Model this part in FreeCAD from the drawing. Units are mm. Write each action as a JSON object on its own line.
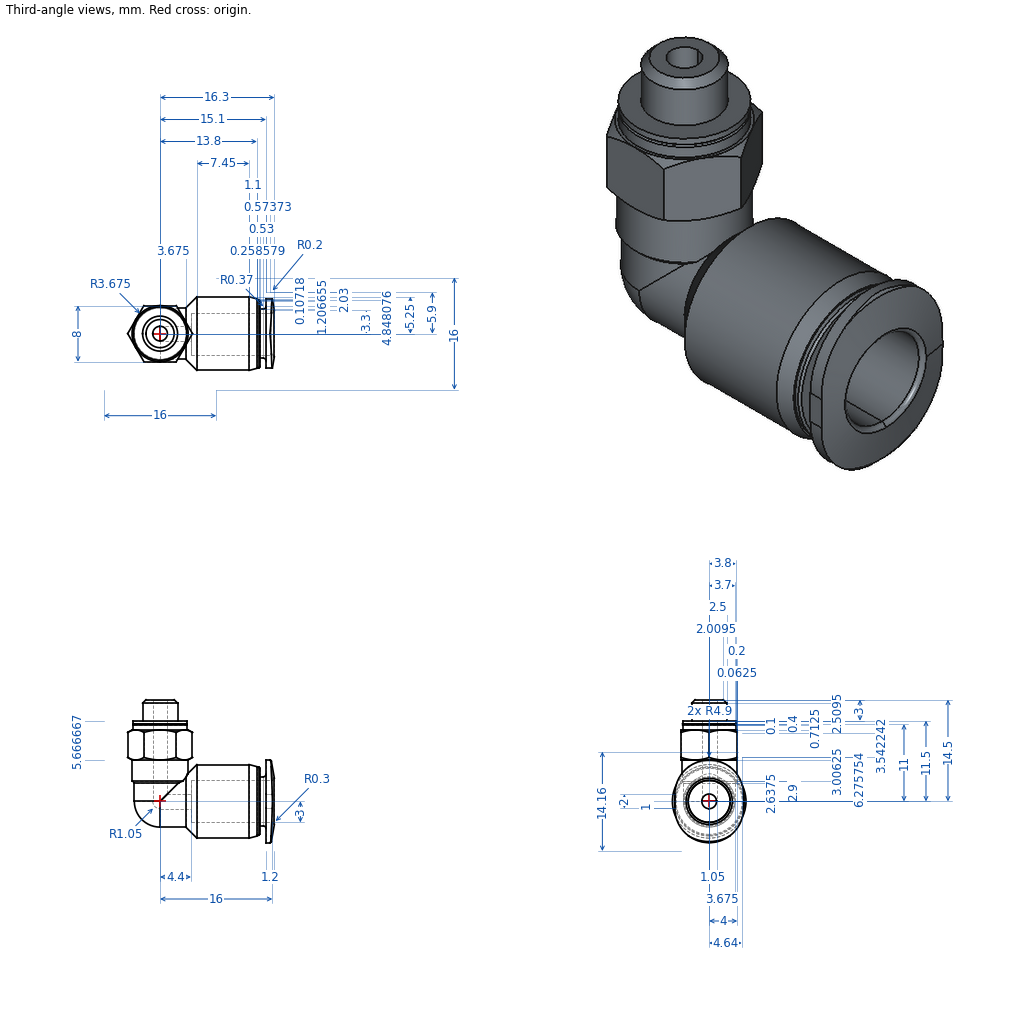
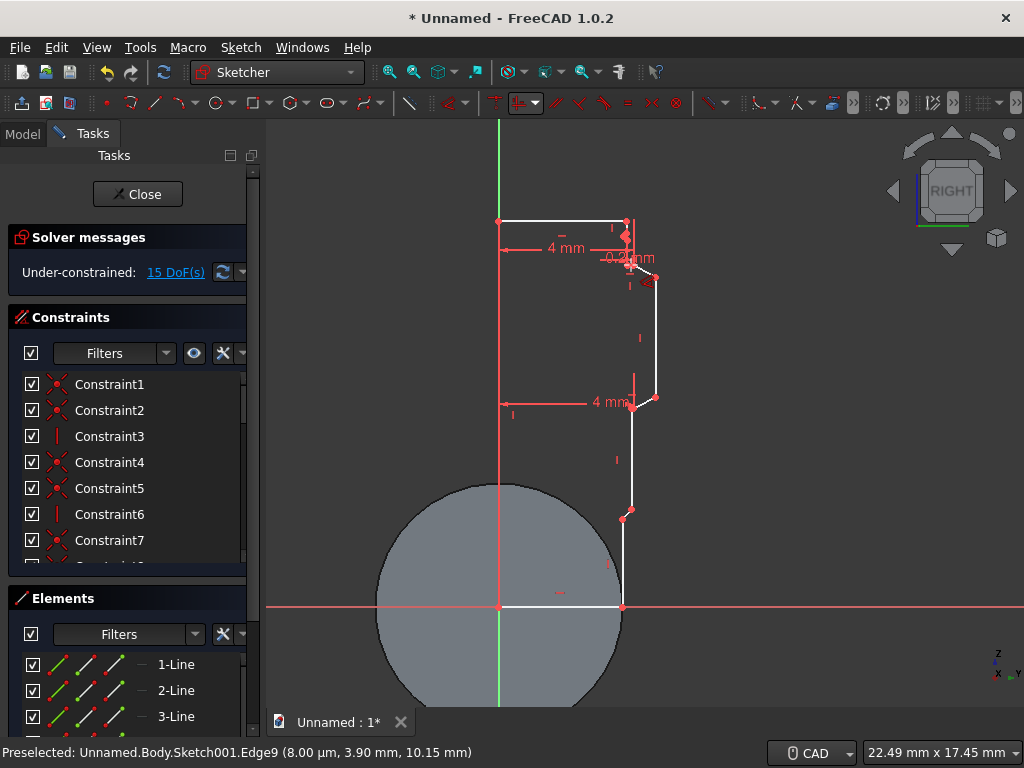
{"action": "scroll", "coordinate": [627, 230], "scroll_direction": "up", "scroll_amount": 7}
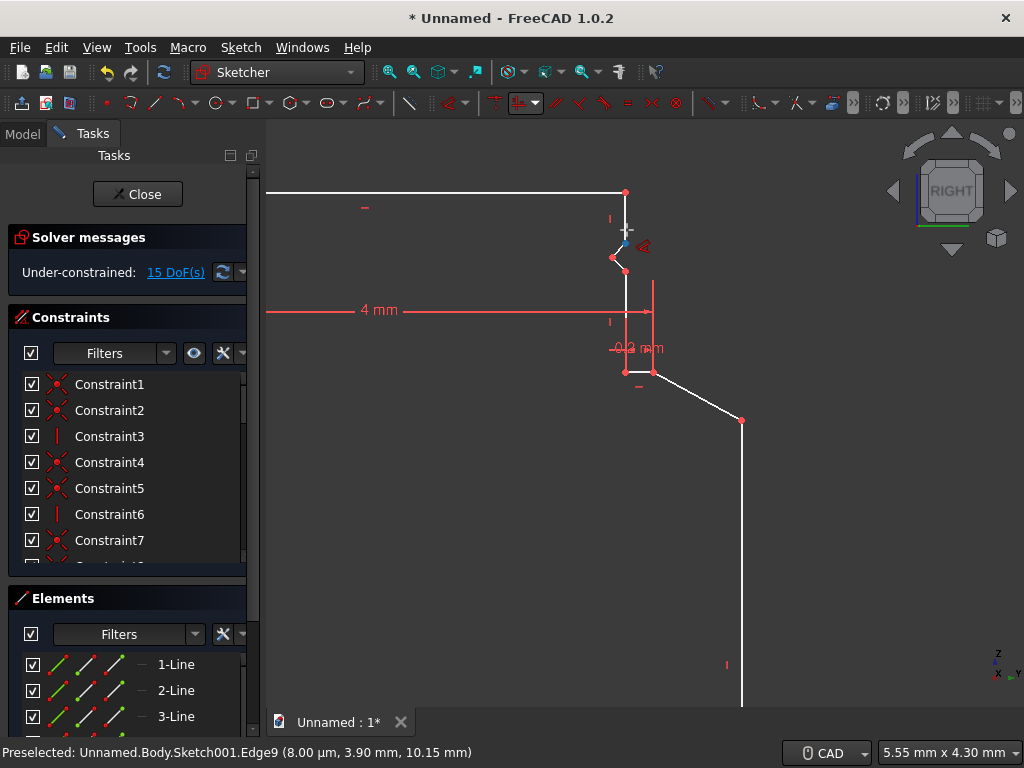
{"action": "left_click", "coordinate": [625, 228]}
{"action": "left_click", "coordinate": [659, 218]}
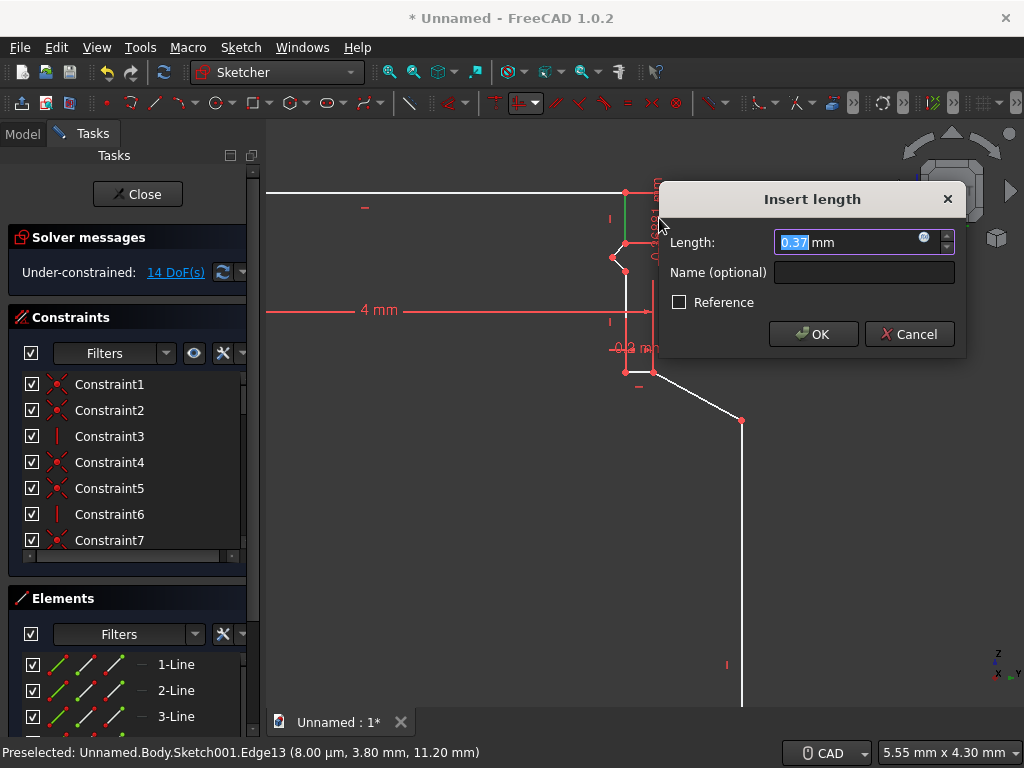
{"action": "type", "text": "0.4"}
{"action": "key", "text": "Return"}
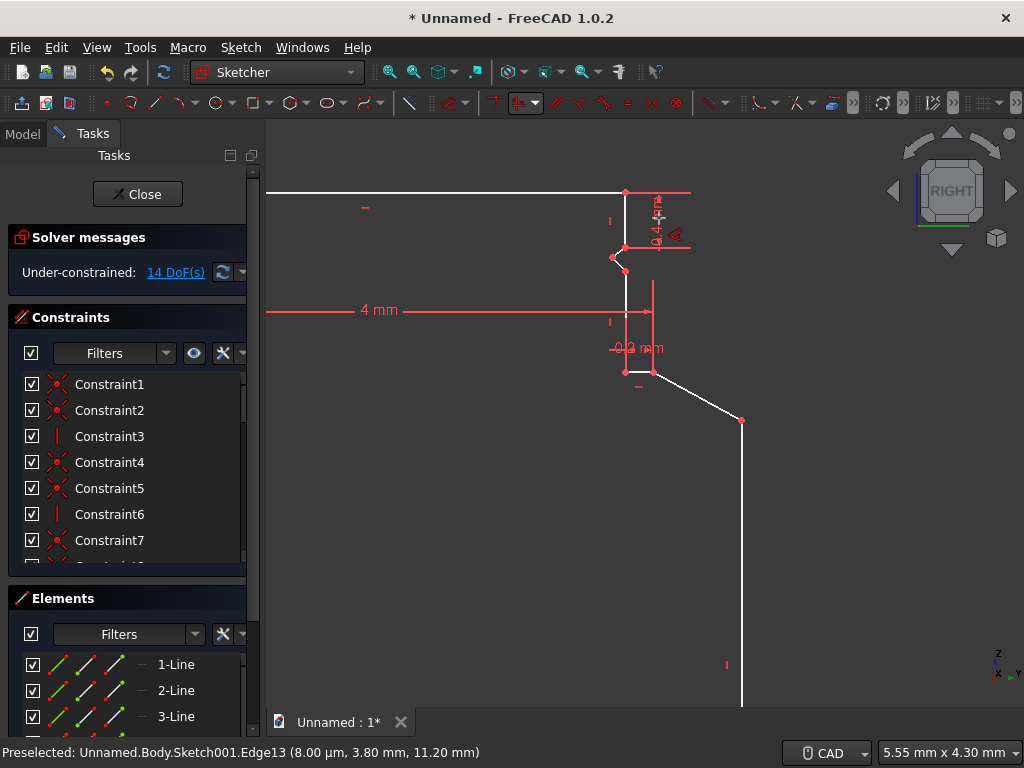
{"action": "scroll", "coordinate": [627, 230], "scroll_direction": "down", "scroll_amount": 7}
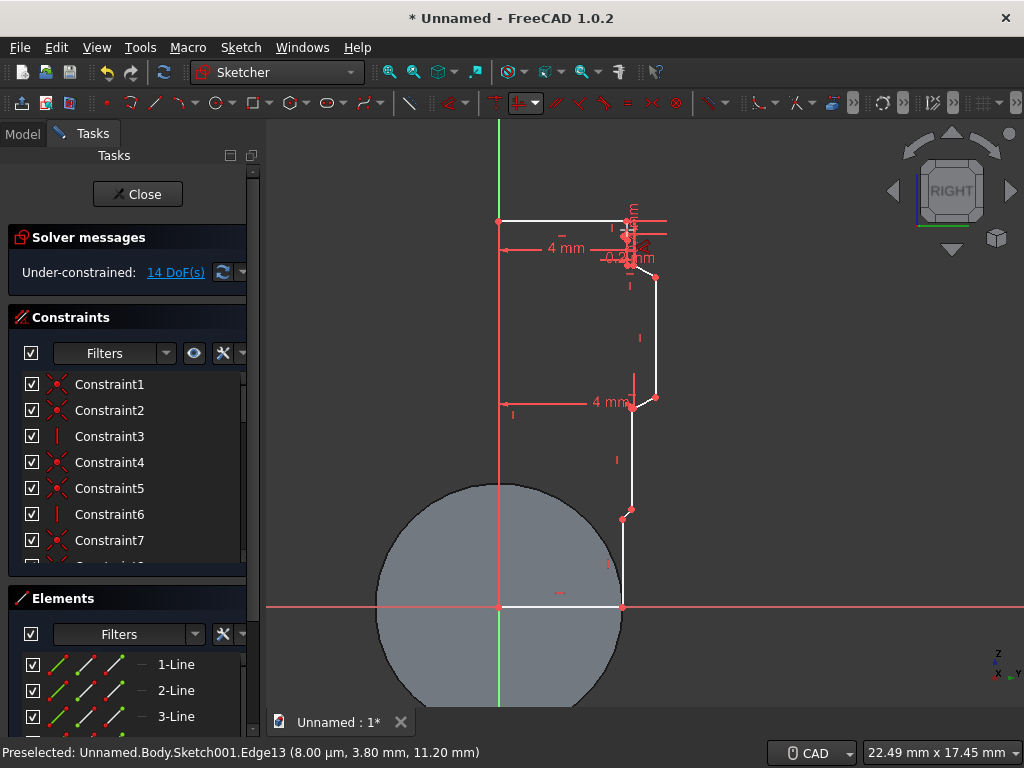
{"action": "left_click", "coordinate": [589, 221]}
{"action": "left_click", "coordinate": [563, 187]}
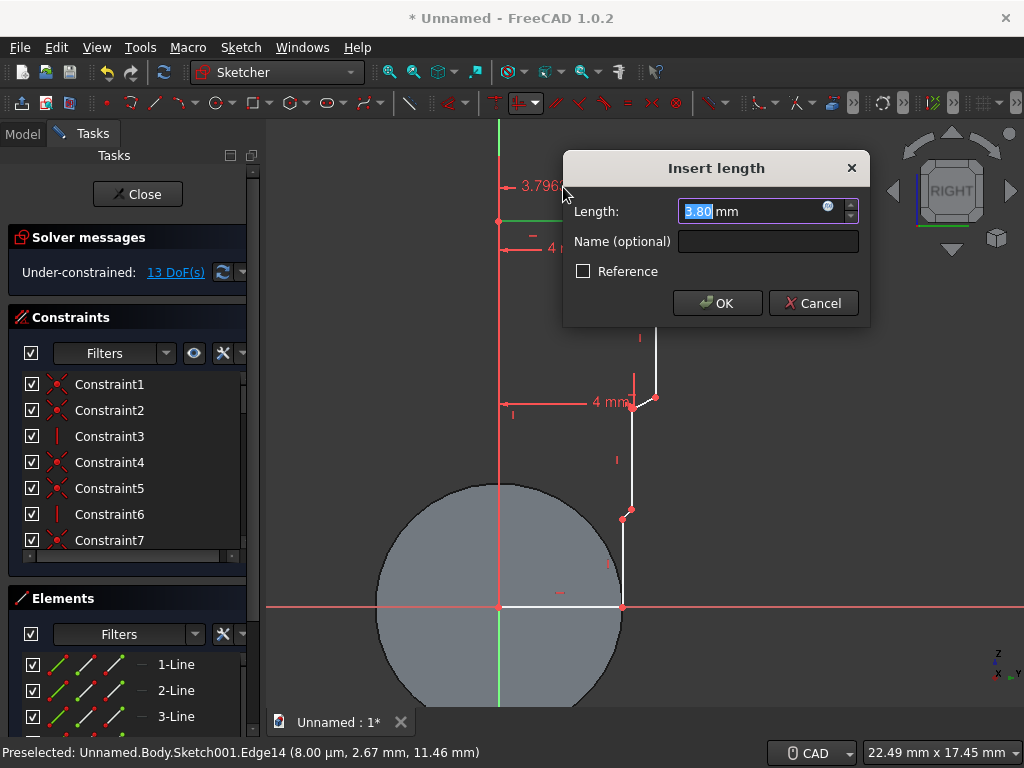
{"action": "type", "text": "3.8"}
{"action": "key", "text": "Return"}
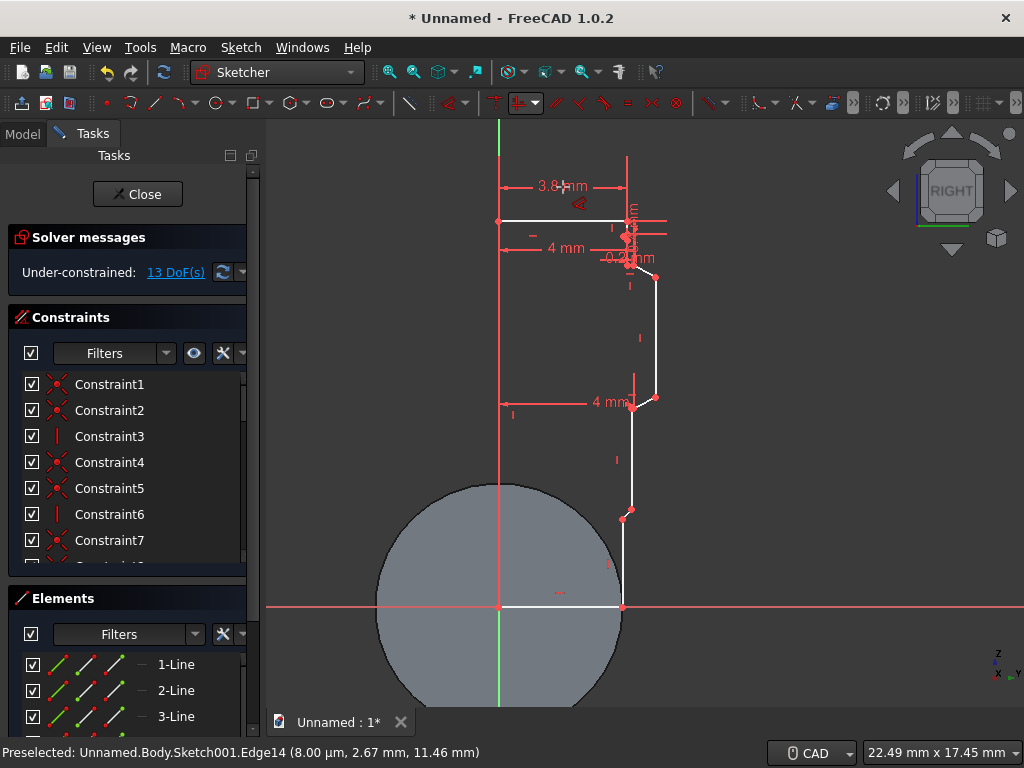
{"action": "scroll", "coordinate": [624, 237], "scroll_direction": "up", "scroll_amount": 6}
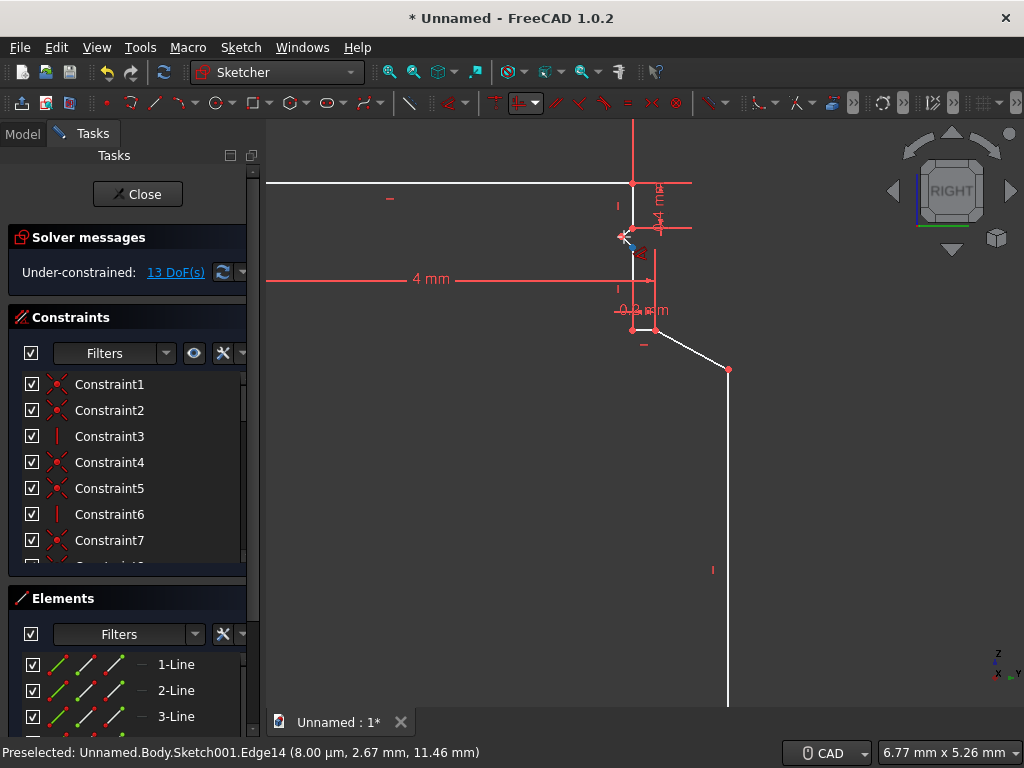
{"action": "left_click", "coordinate": [622, 236]}
{"action": "left_click", "coordinate": [656, 458]}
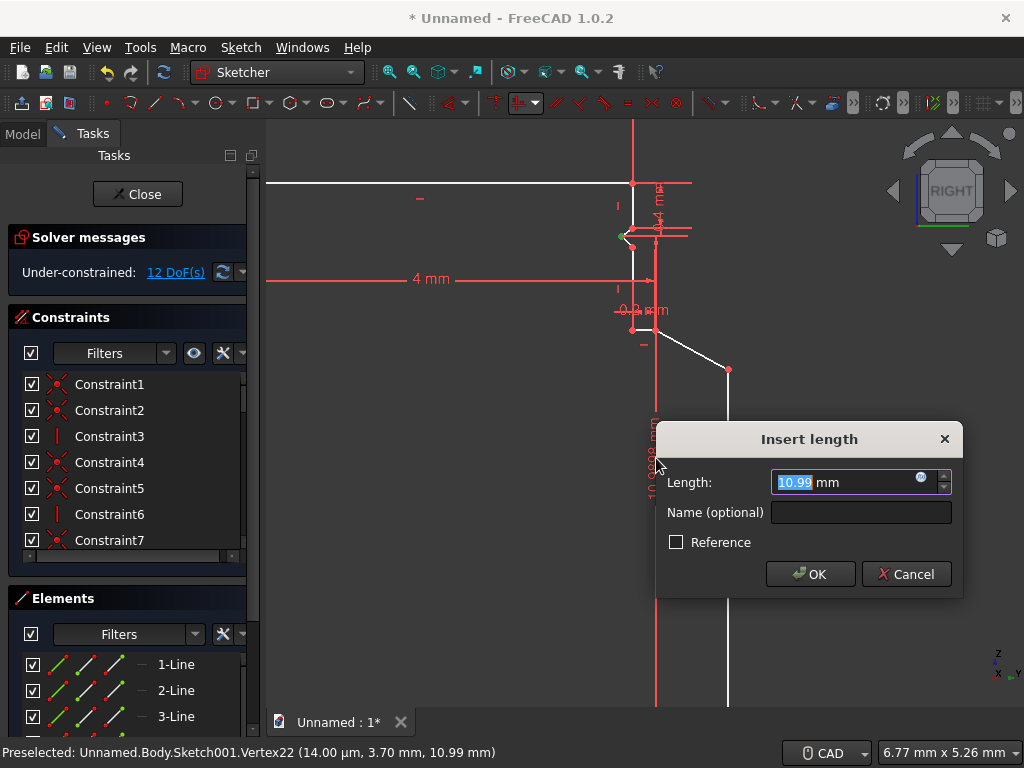
{"action": "type", "text": "11"}
{"action": "key", "text": "Return"}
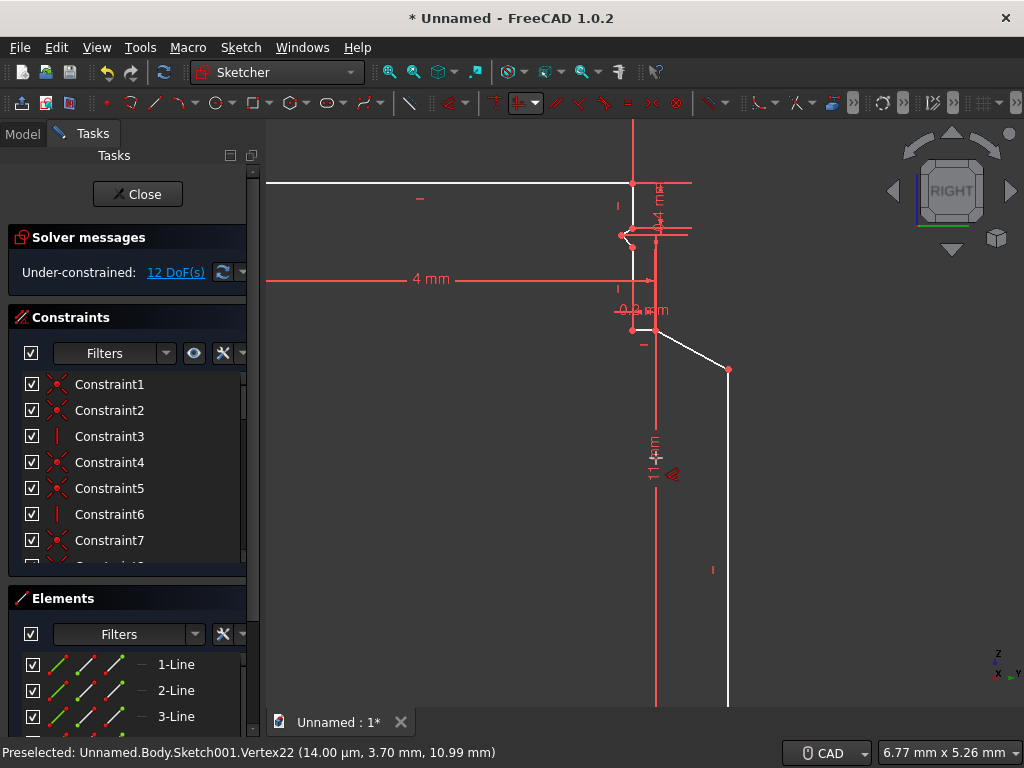
{"action": "scroll", "coordinate": [624, 237], "scroll_direction": "down", "scroll_amount": 6}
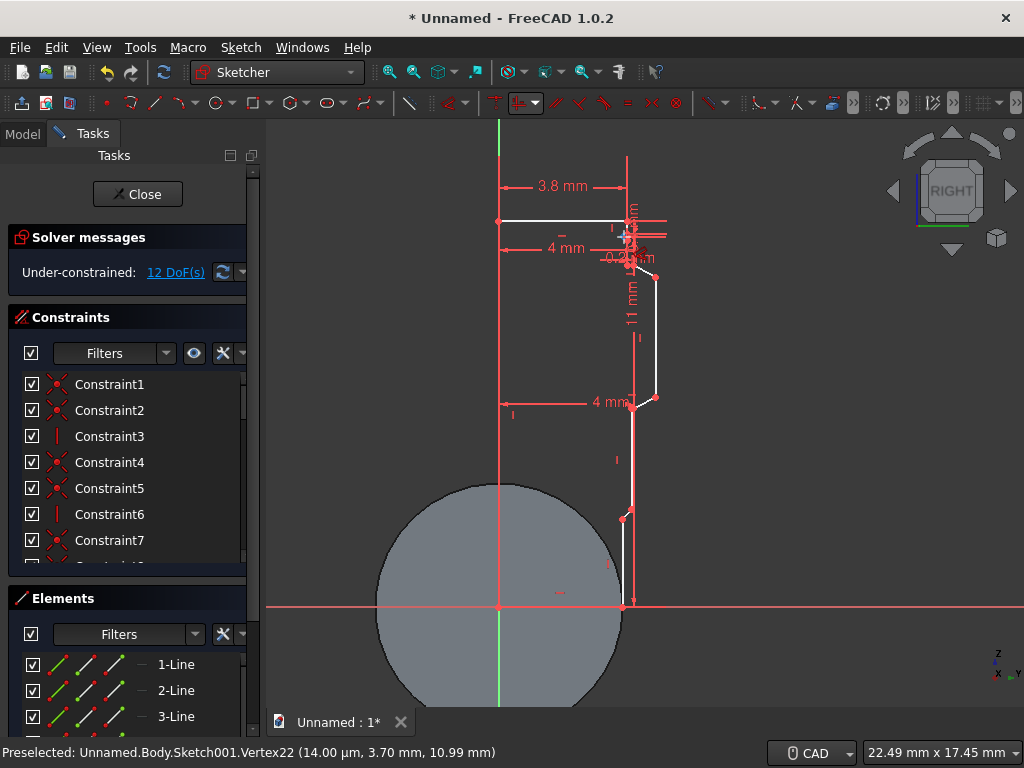
{"action": "left_click", "coordinate": [499, 337]}
{"action": "left_click", "coordinate": [465, 414]}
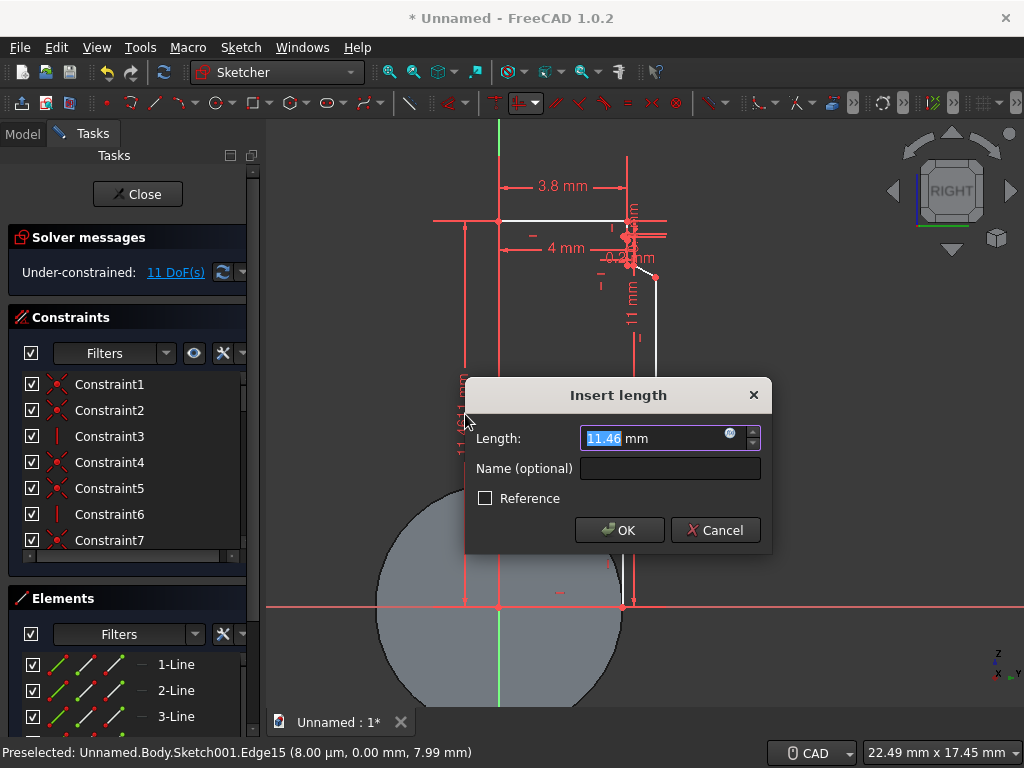
{"action": "type", "text": "11.5"}
{"action": "key", "text": "Return"}